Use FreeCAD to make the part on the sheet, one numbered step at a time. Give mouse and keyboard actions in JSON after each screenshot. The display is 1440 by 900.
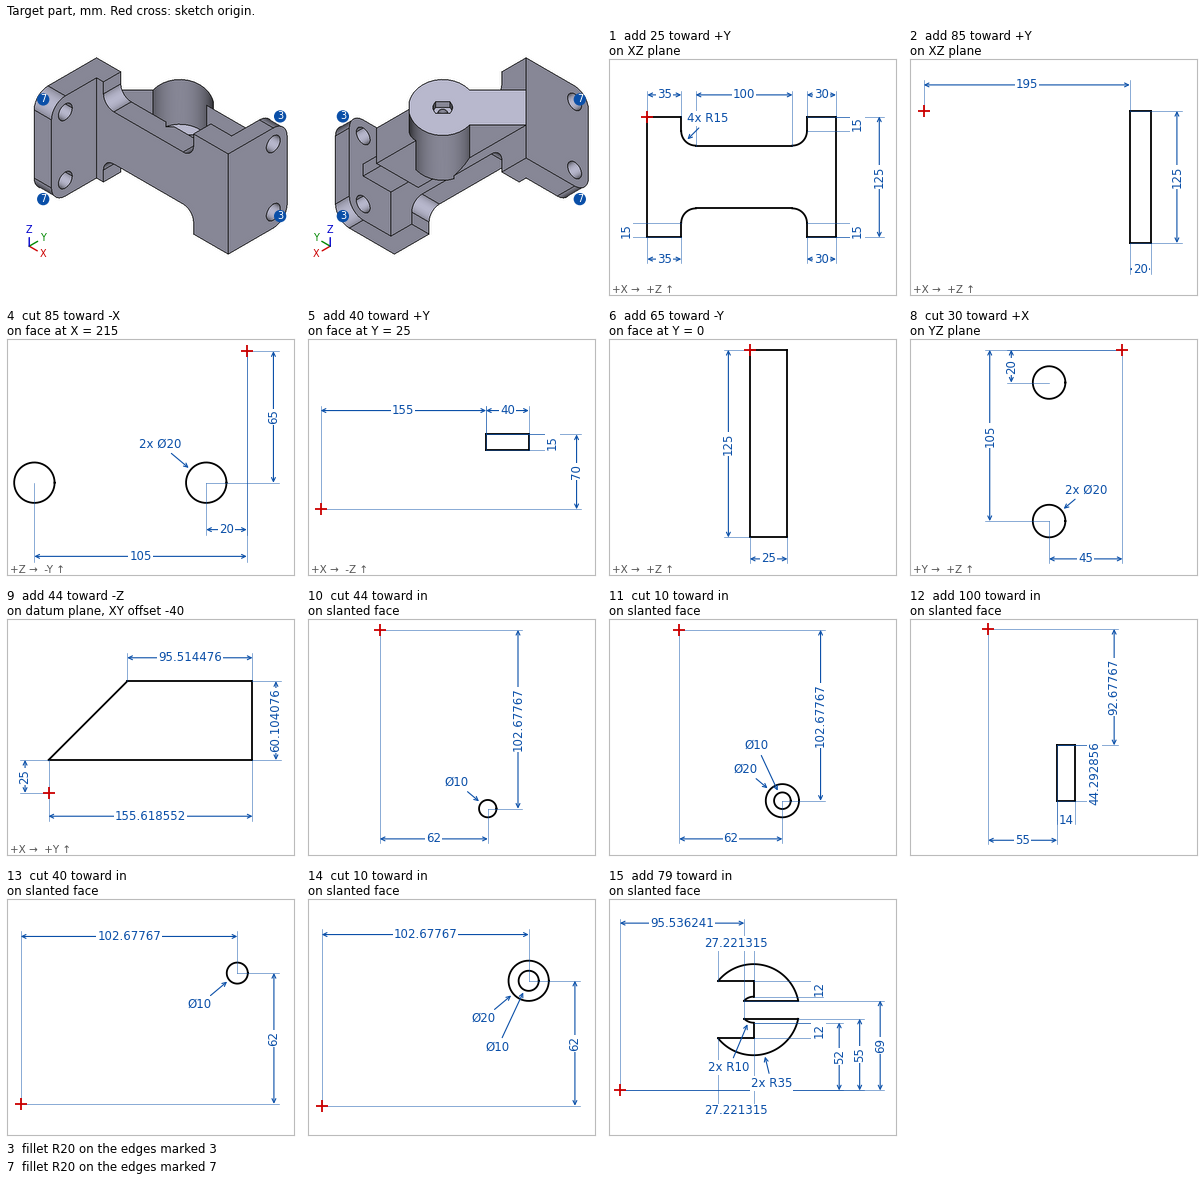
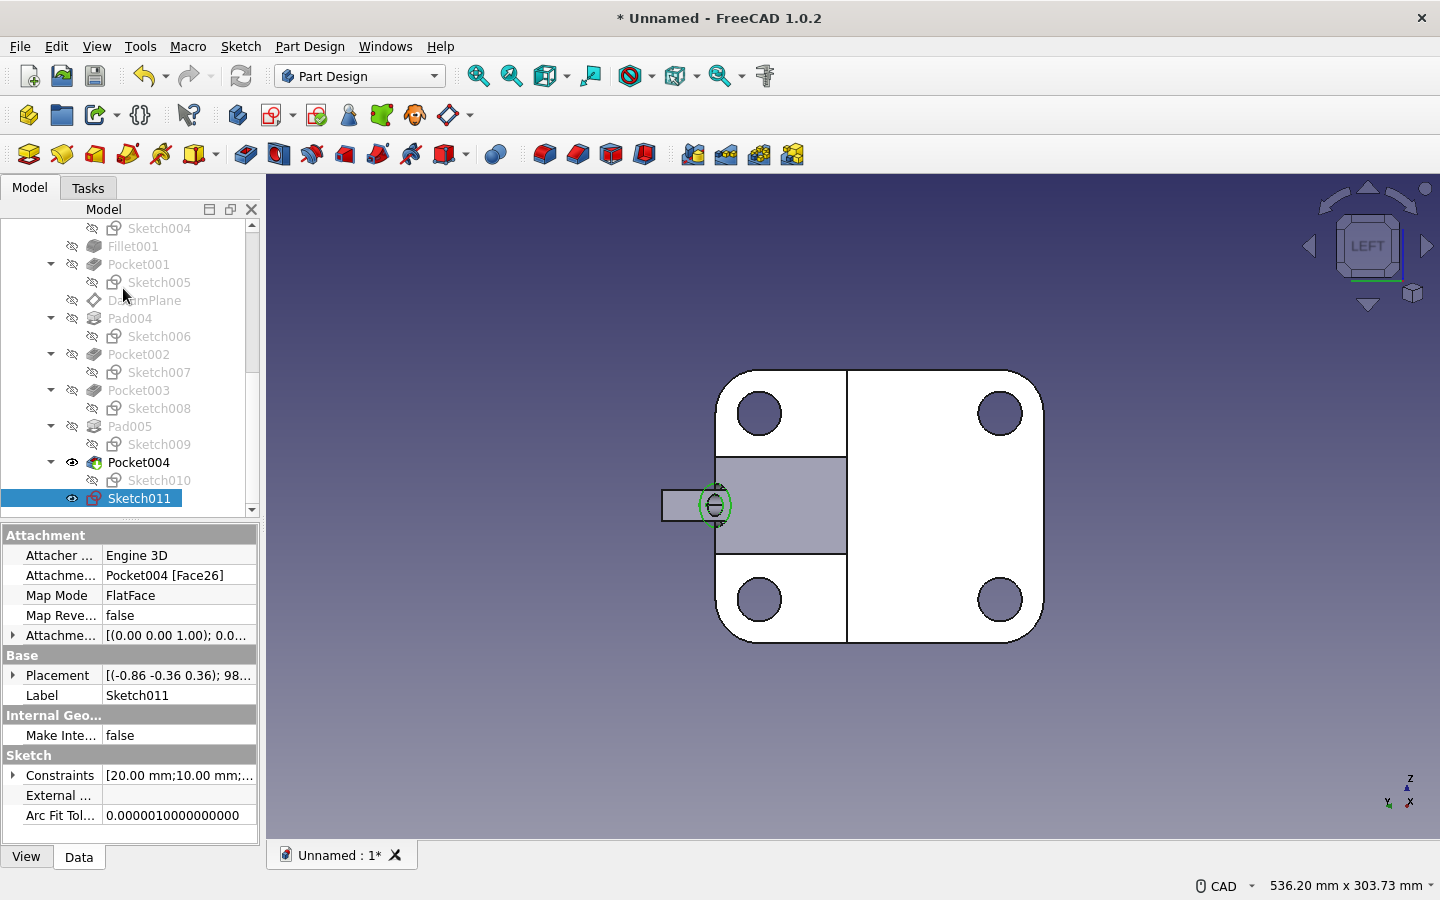
{"action": "left_click", "coordinate": [246, 154]}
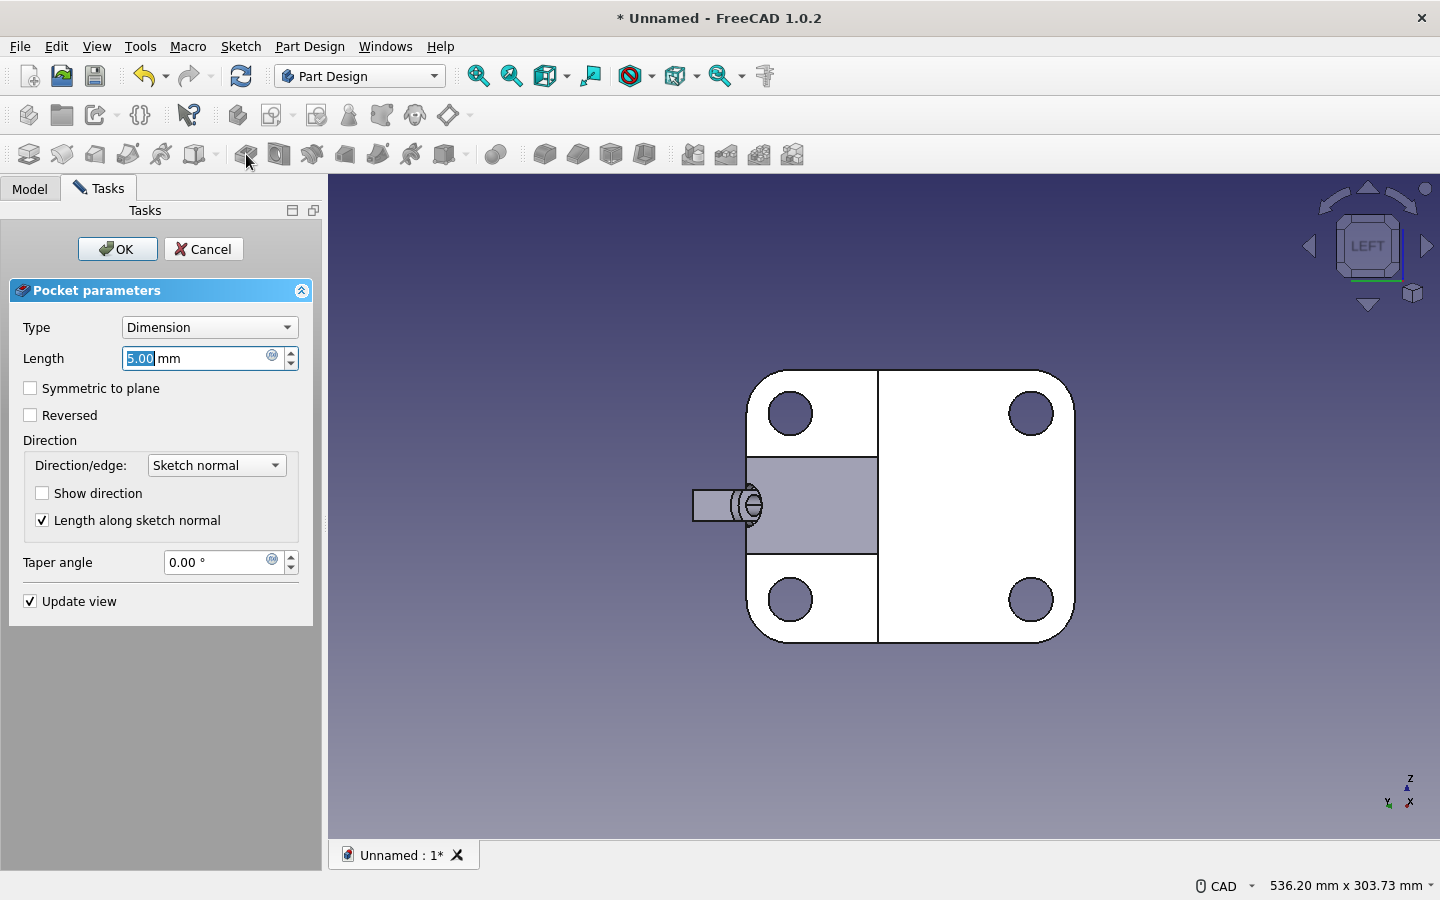
{"action": "type", "text": "10"}
{"action": "key", "text": "Tab"}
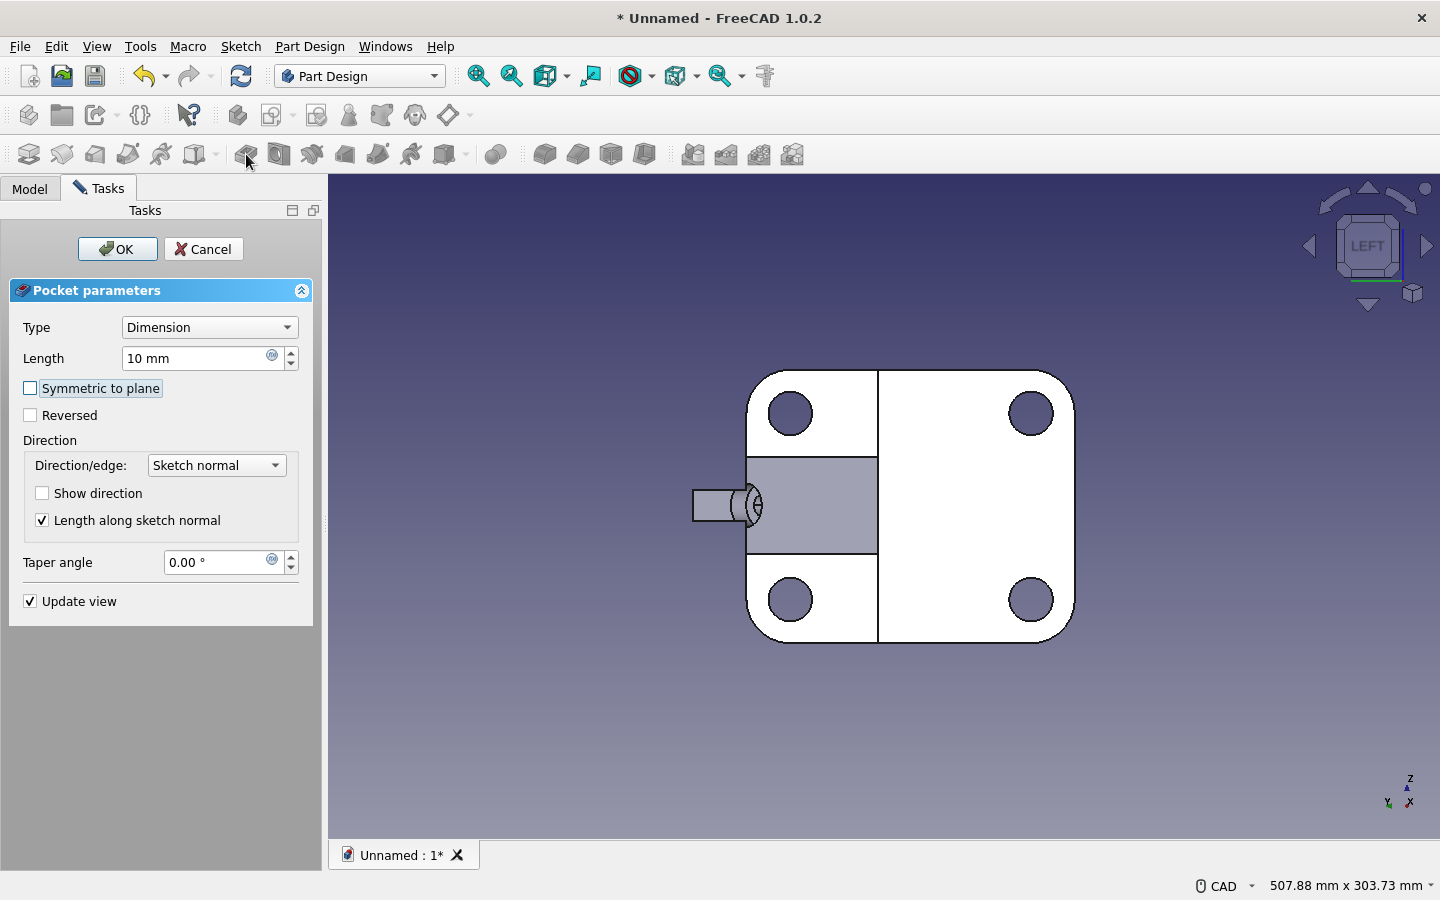
{"action": "left_click", "coordinate": [118, 249]}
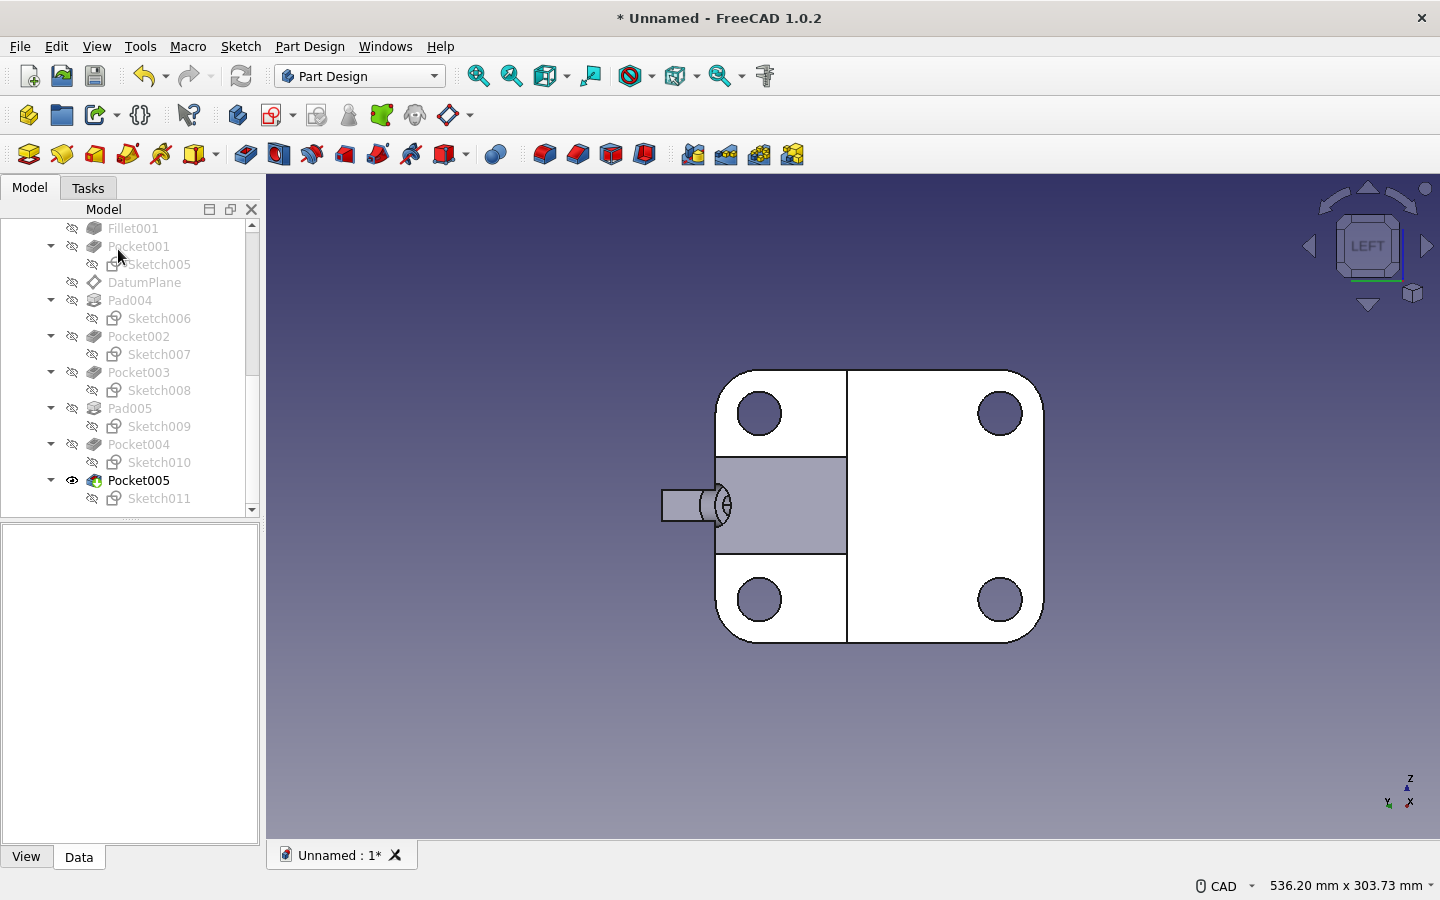
{"action": "left_click", "coordinate": [479, 76]}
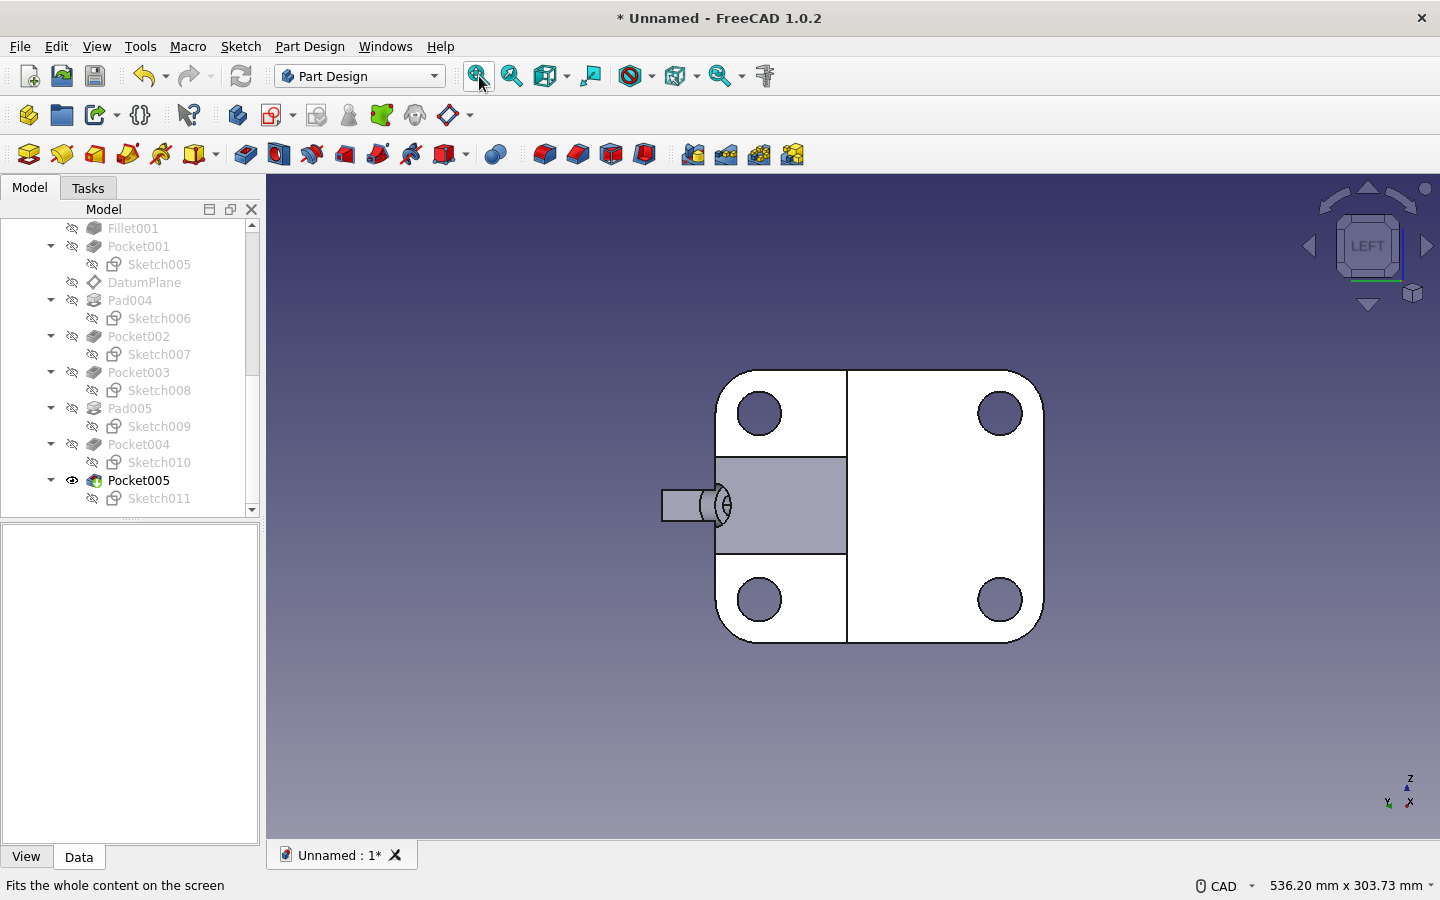
{"action": "left_click", "coordinate": [781, 504]}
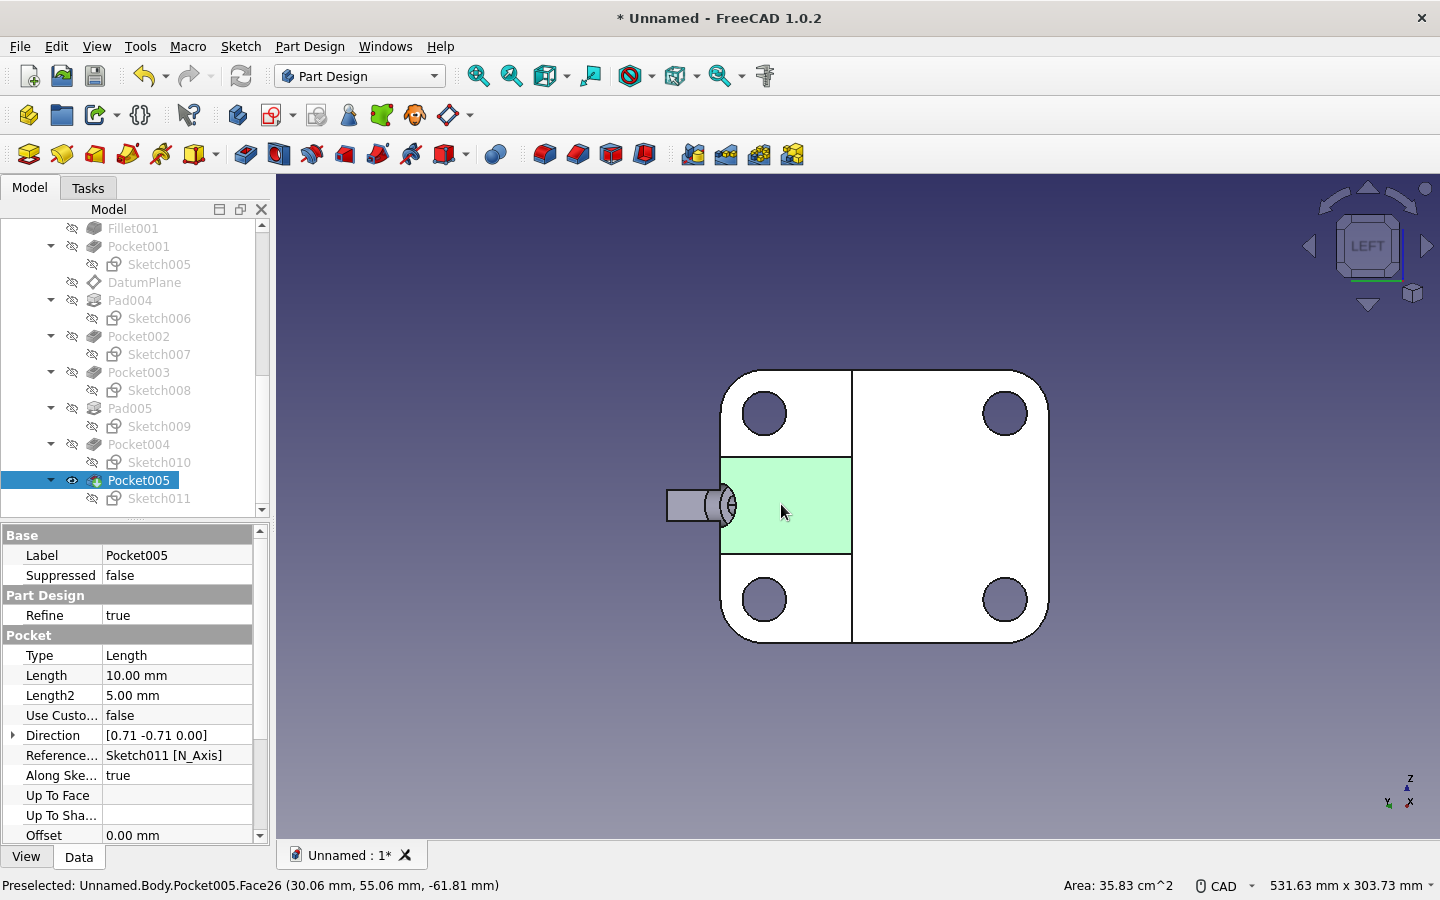
{"action": "left_click", "coordinate": [270, 116]}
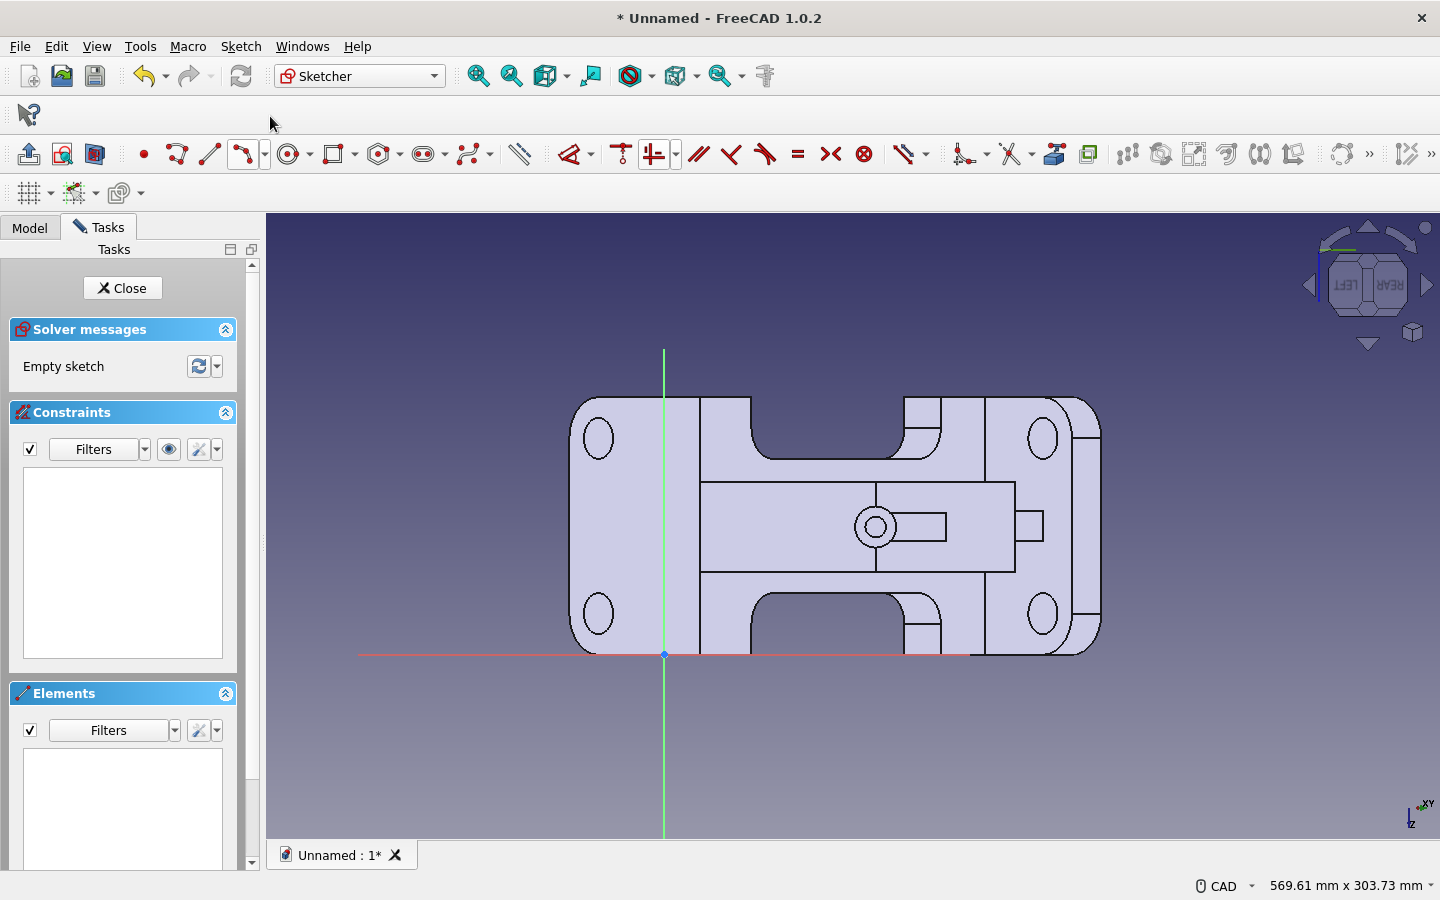
{"action": "key", "text": "q s"}